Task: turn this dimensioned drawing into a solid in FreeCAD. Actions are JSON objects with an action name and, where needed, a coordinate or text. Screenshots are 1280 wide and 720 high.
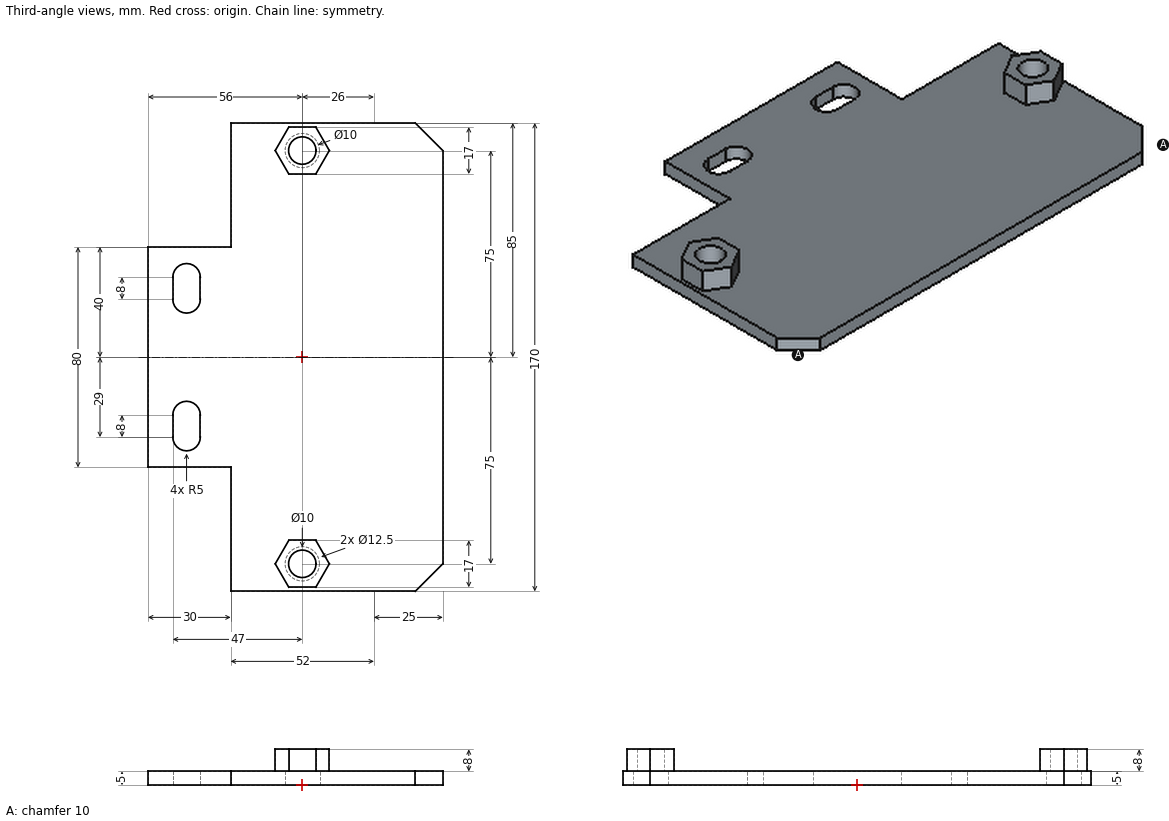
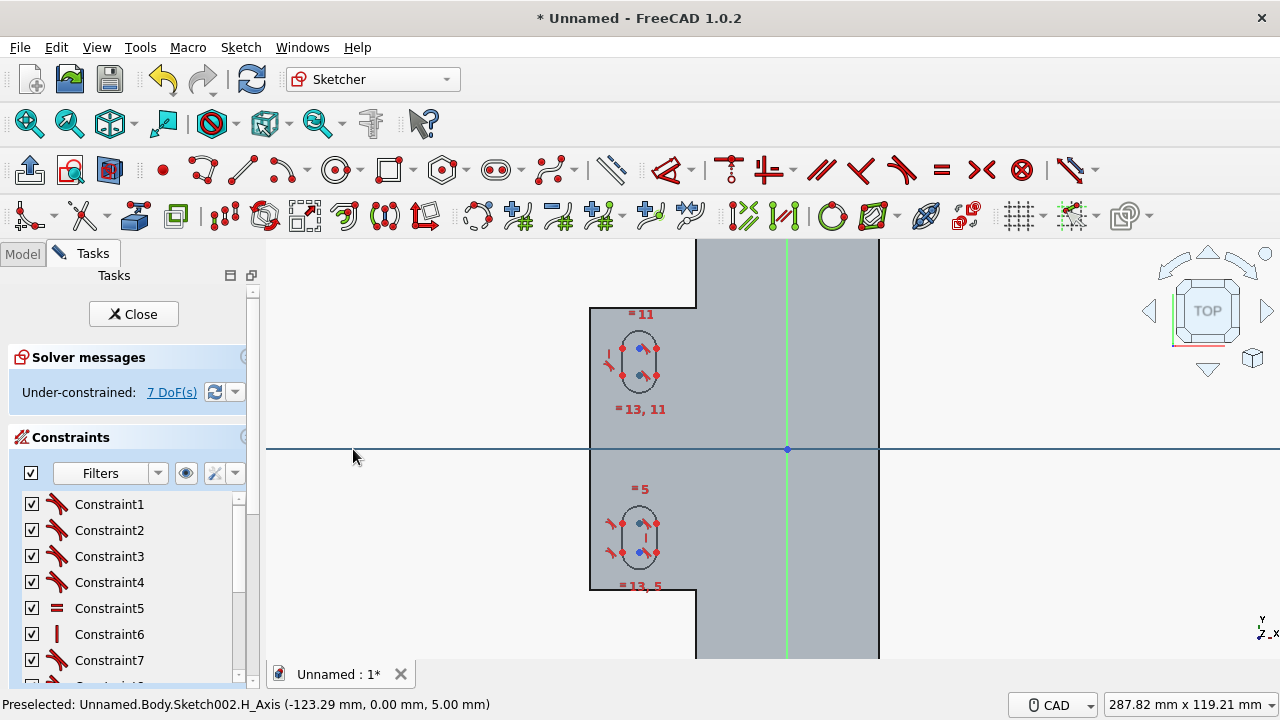
{"action": "left_click", "coordinate": [982, 170]}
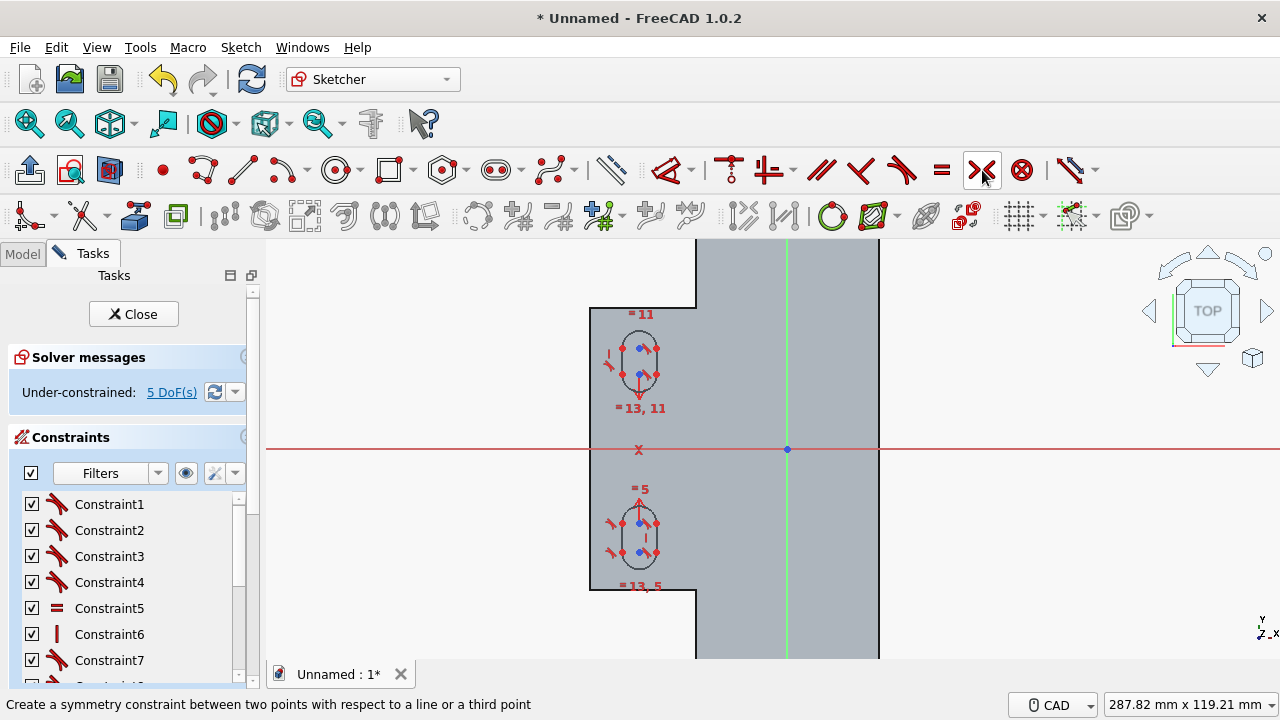
{"action": "left_click", "coordinate": [666, 170]}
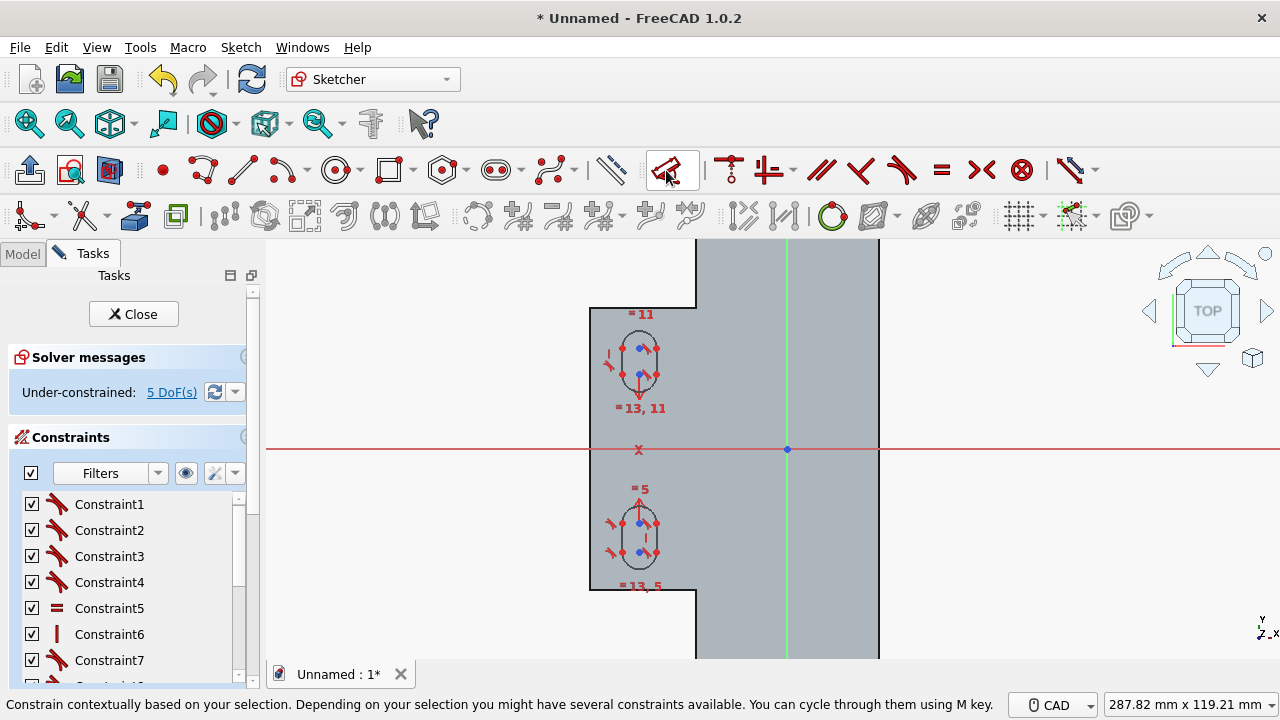
{"action": "scroll", "coordinate": [629, 566], "scroll_direction": "up", "scroll_amount": 5}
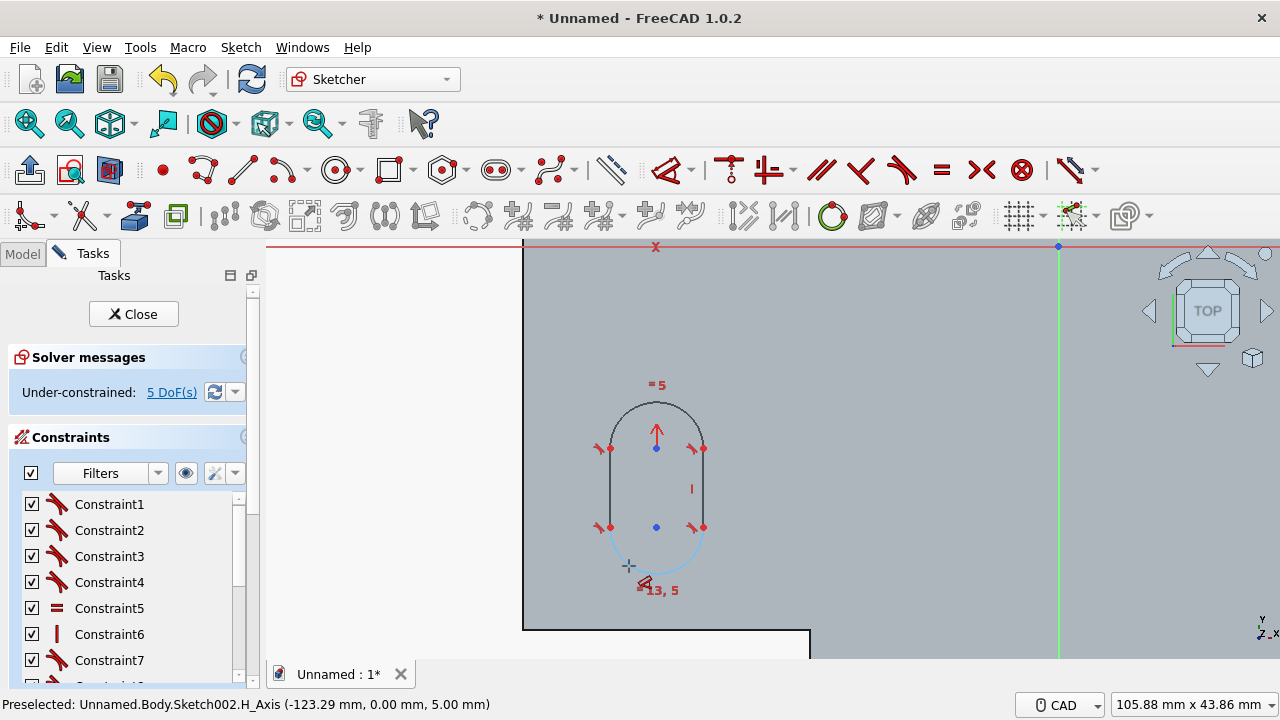
{"action": "left_click", "coordinate": [629, 565]}
{"action": "left_click", "coordinate": [610, 591]}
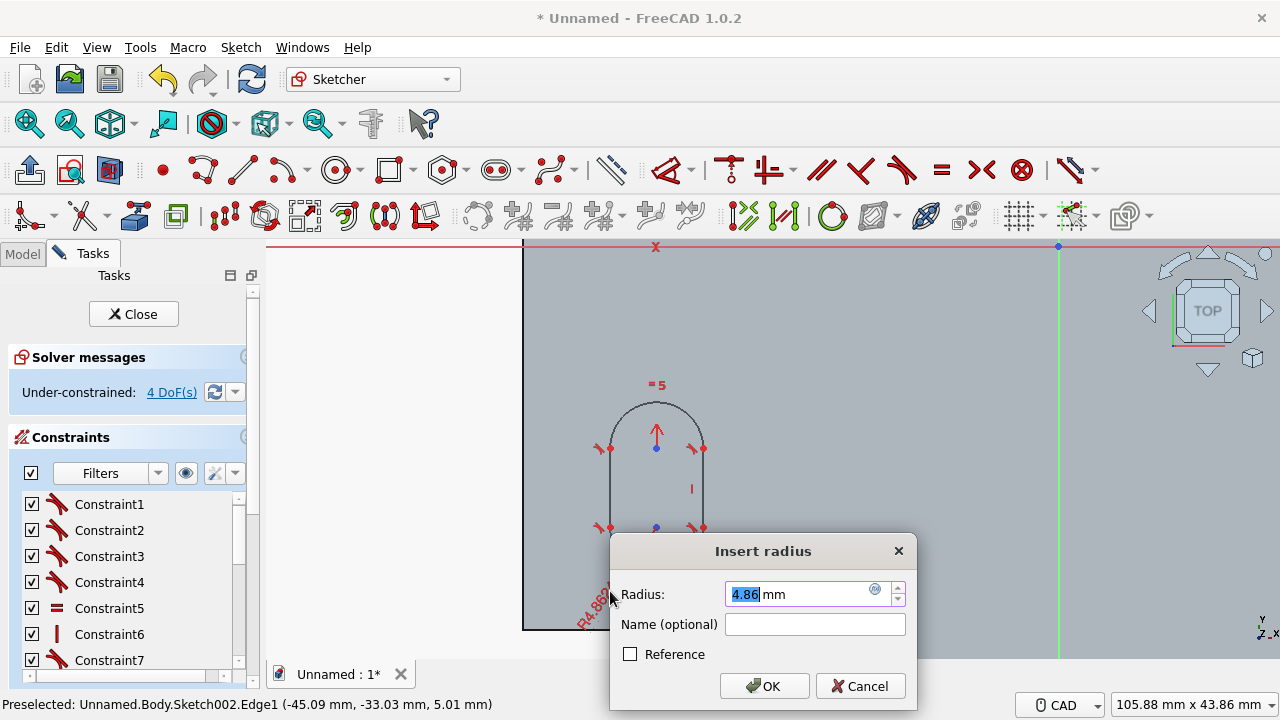
{"action": "type", "text": "5"}
{"action": "key", "text": "Return"}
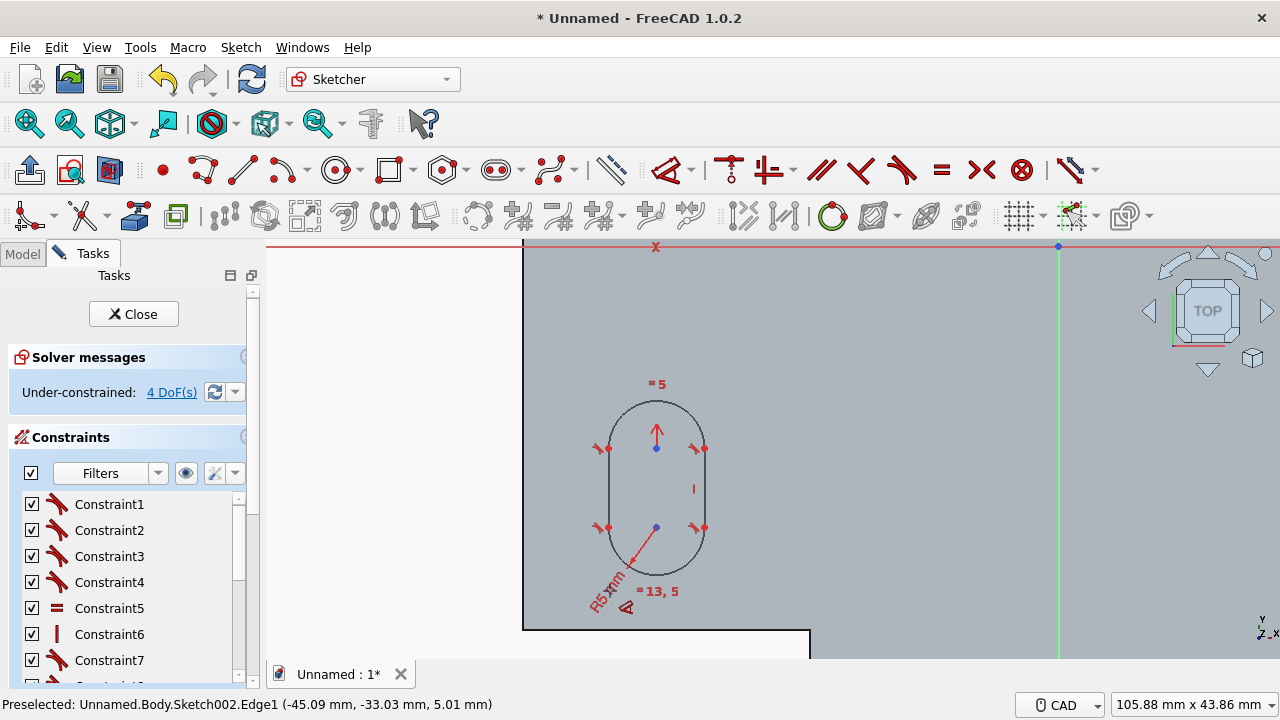
{"action": "left_click", "coordinate": [609, 504]}
{"action": "left_click", "coordinate": [575, 488]}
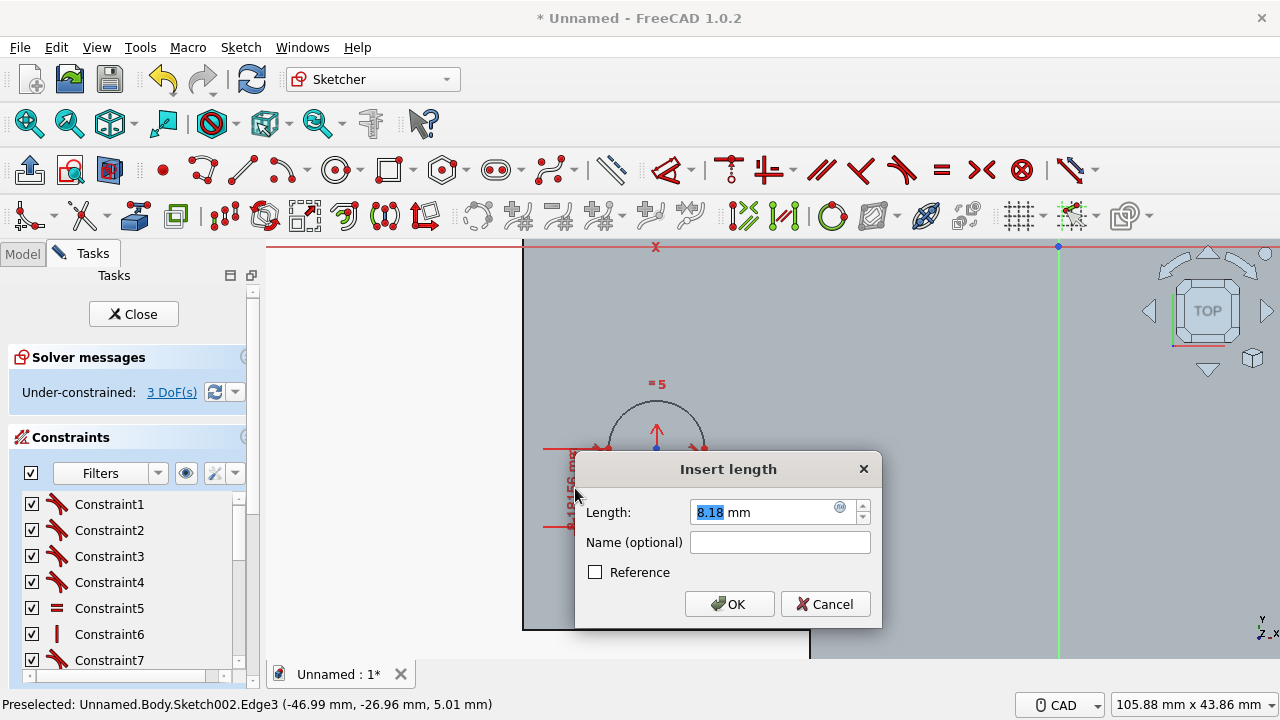
{"action": "type", "text": "8"}
{"action": "key", "text": "Return"}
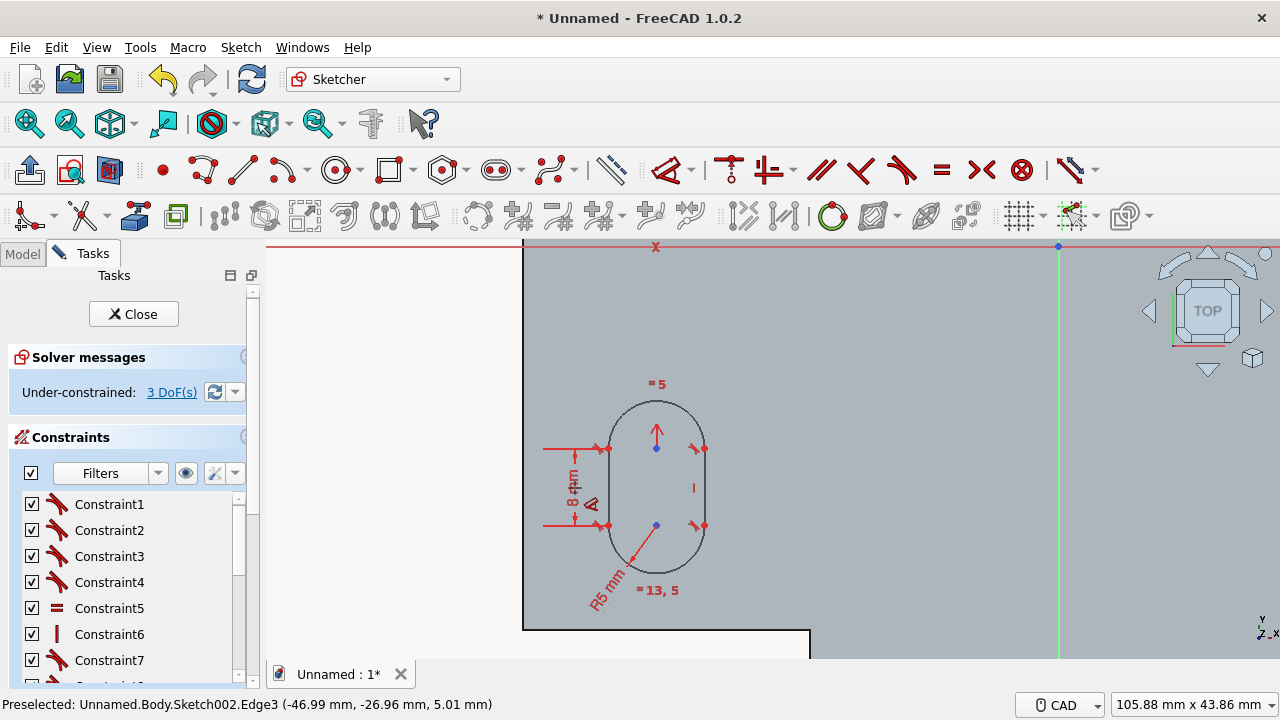
{"action": "scroll", "coordinate": [629, 567], "scroll_direction": "down", "scroll_amount": 5}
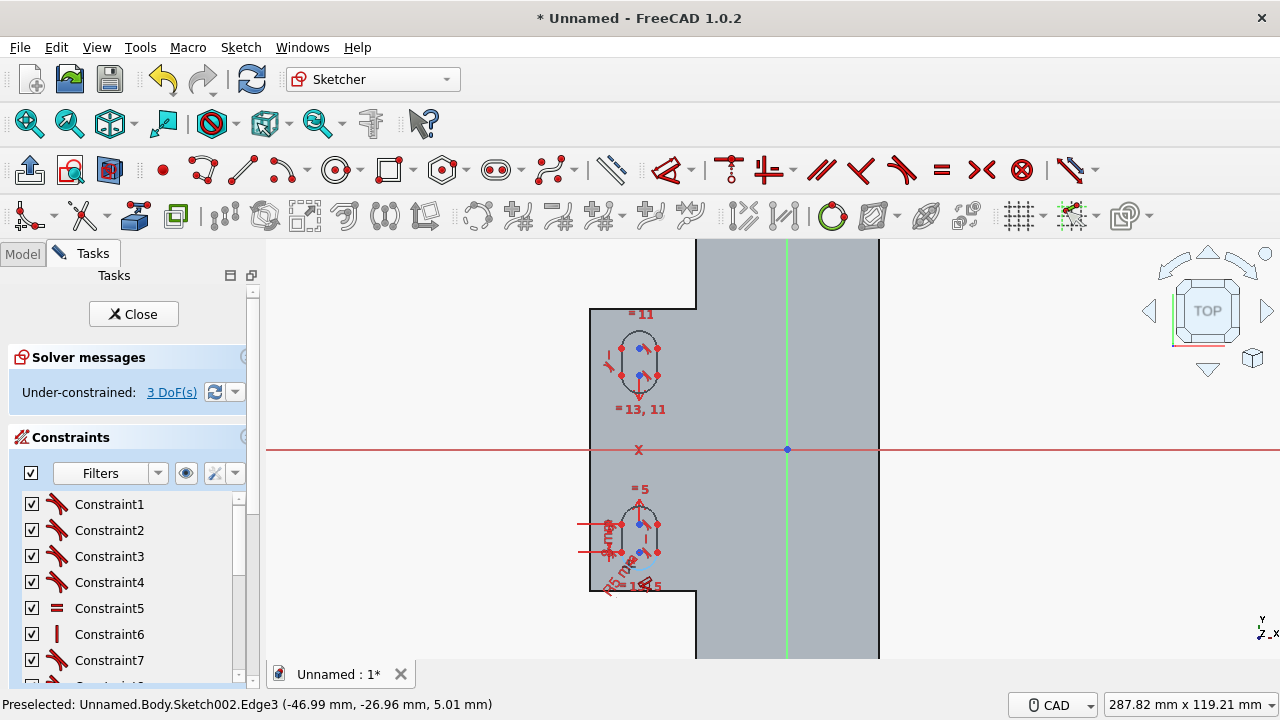
{"action": "scroll", "coordinate": [622, 367], "scroll_direction": "up", "scroll_amount": 3}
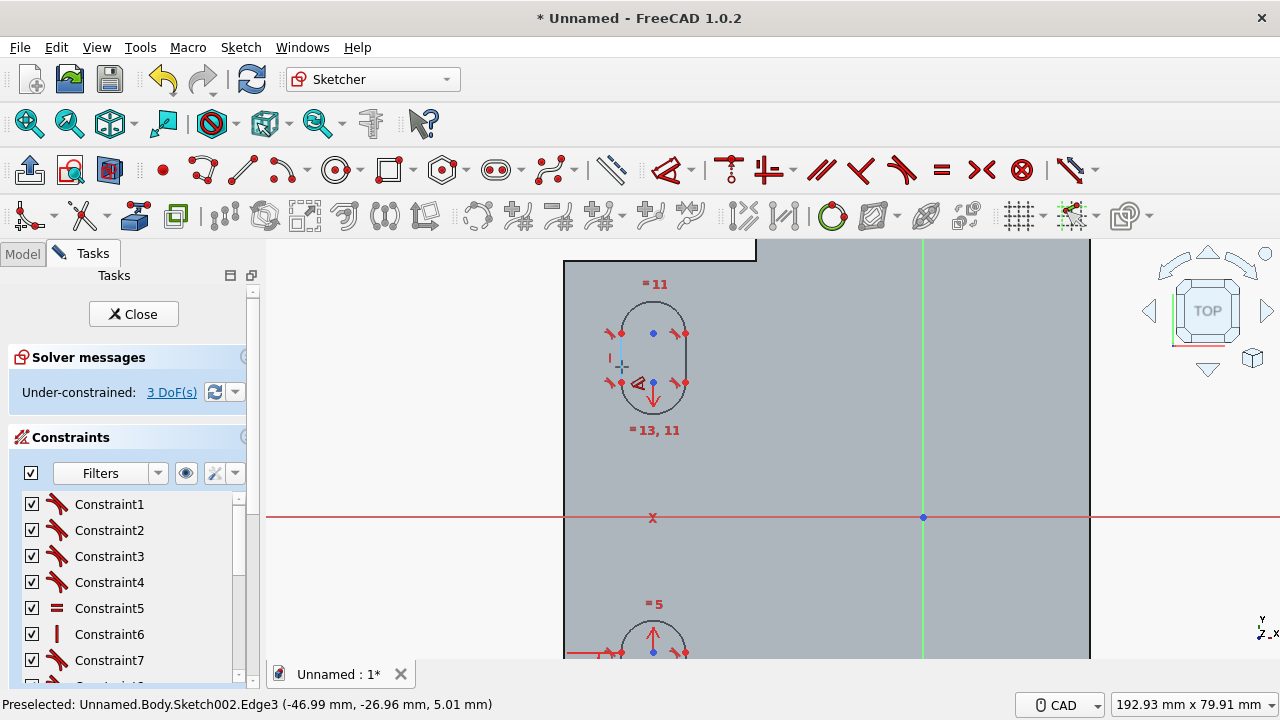
{"action": "left_click", "coordinate": [621, 368]}
{"action": "left_click", "coordinate": [587, 358]}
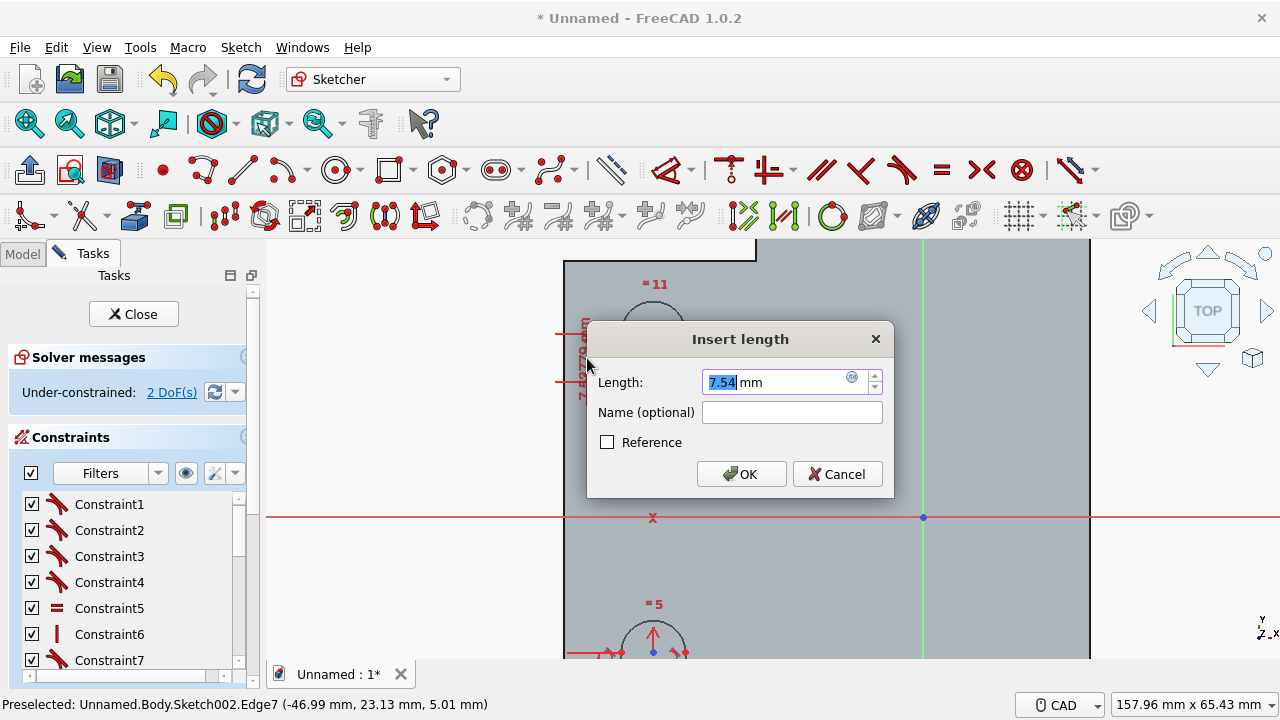
{"action": "type", "text": "8"}
{"action": "key", "text": "Return"}